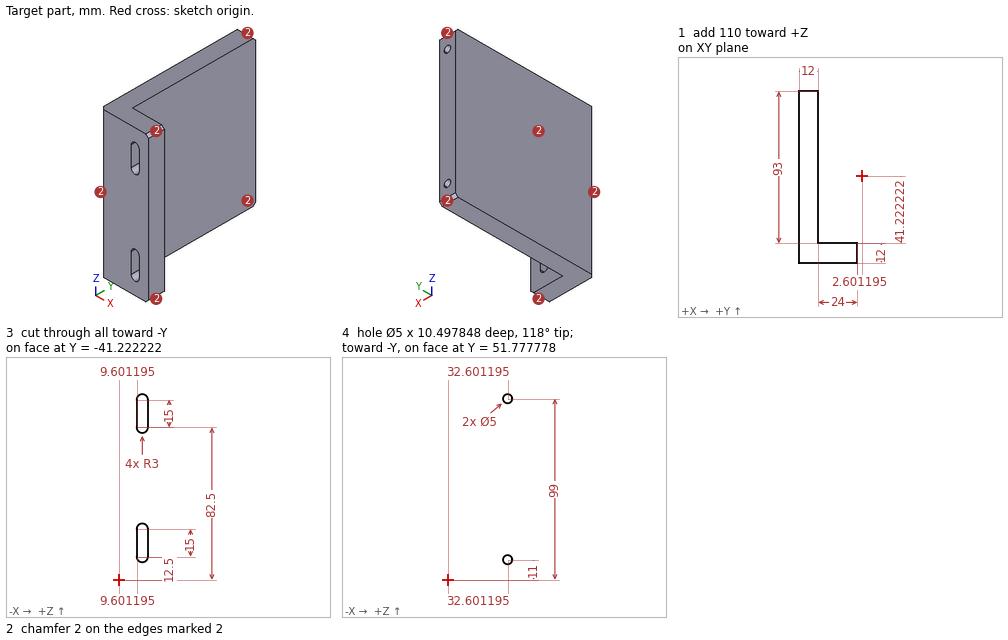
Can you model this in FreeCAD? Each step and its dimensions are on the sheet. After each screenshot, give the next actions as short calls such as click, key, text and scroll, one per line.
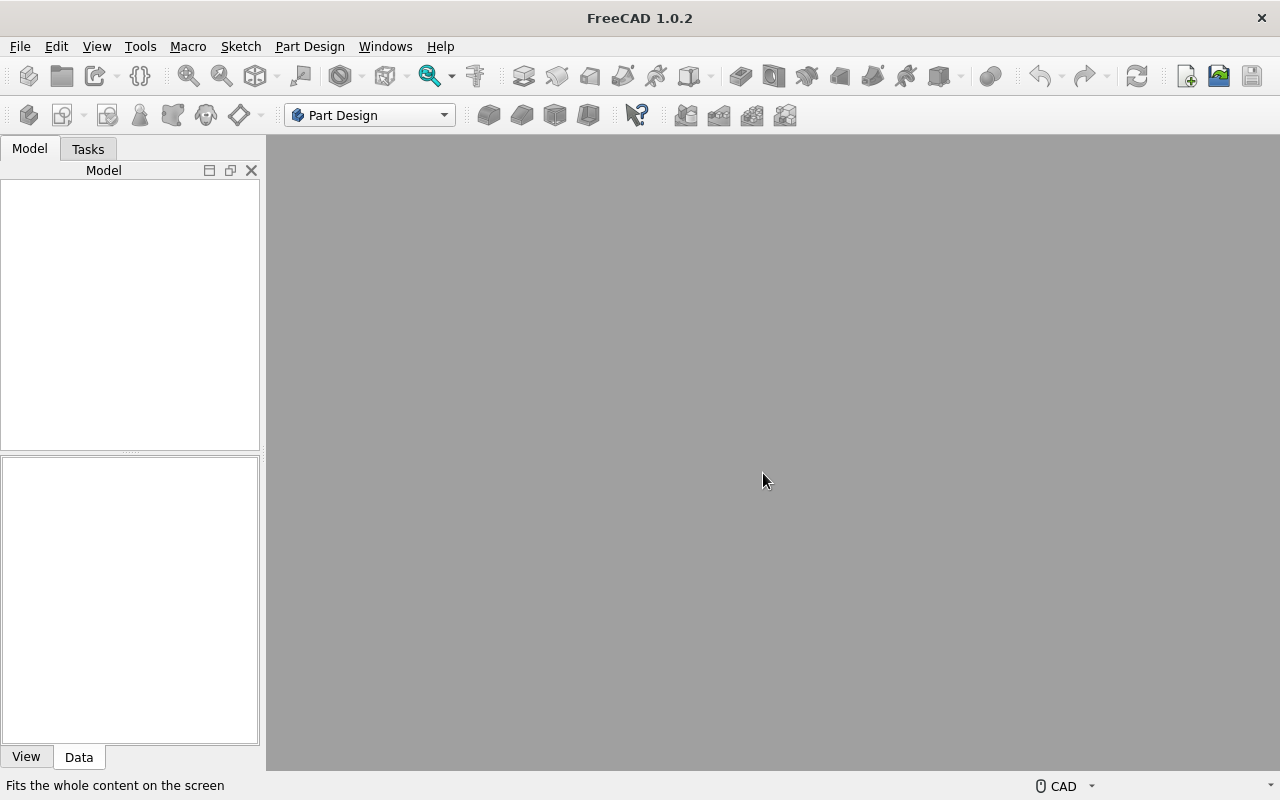
click(1186, 76)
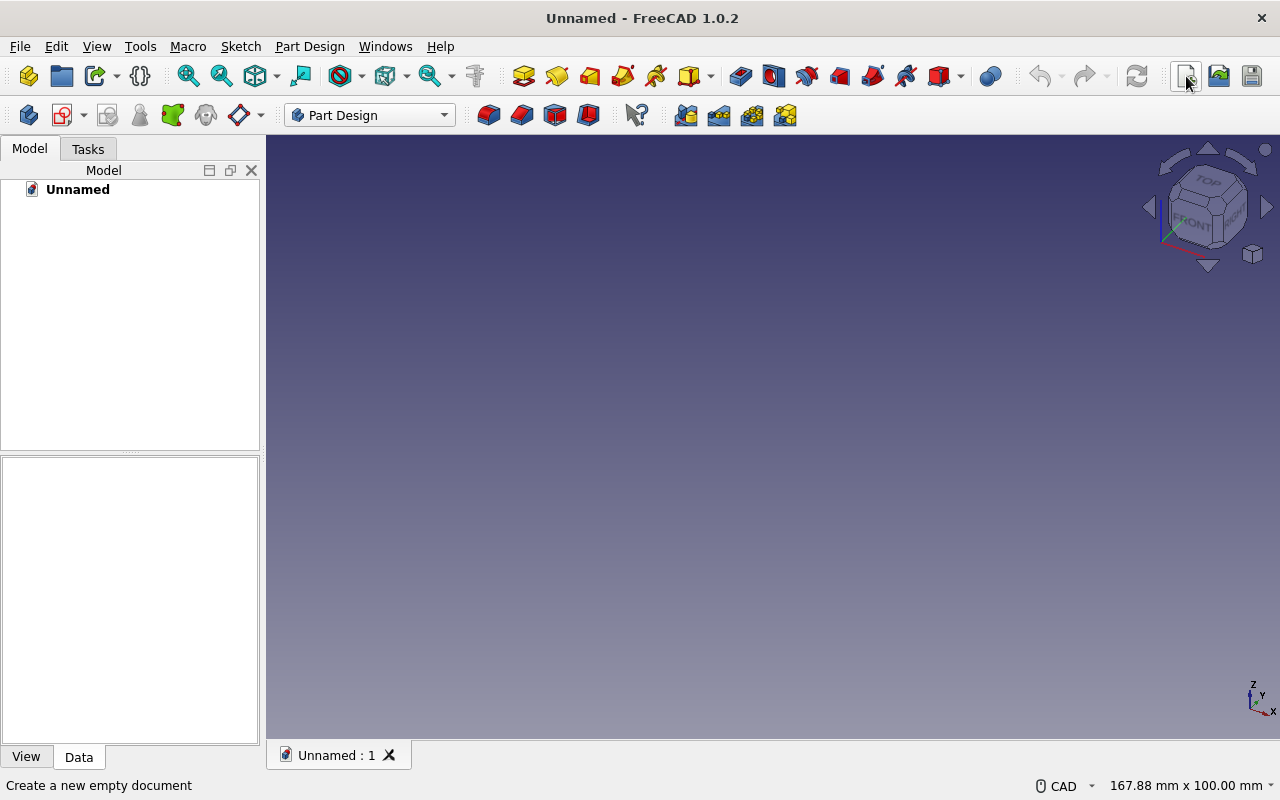
click(62, 116)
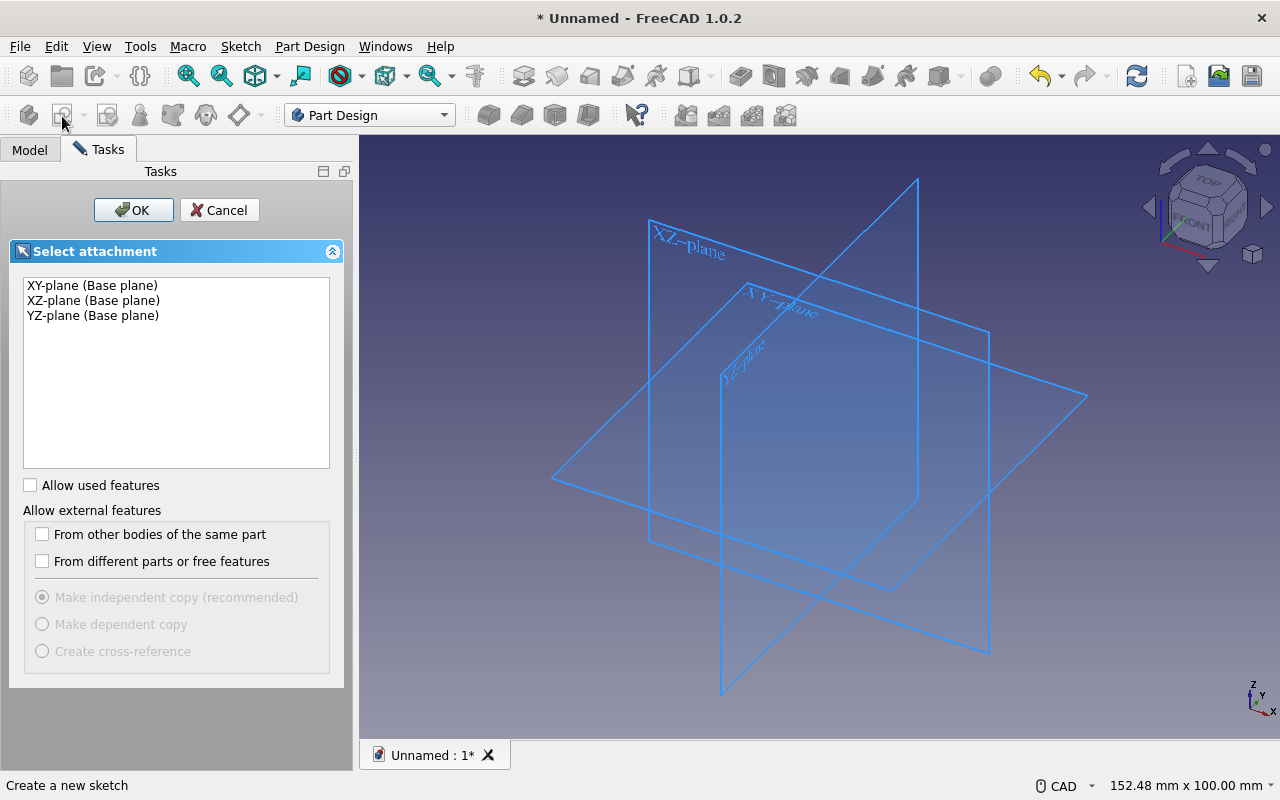
click(84, 286)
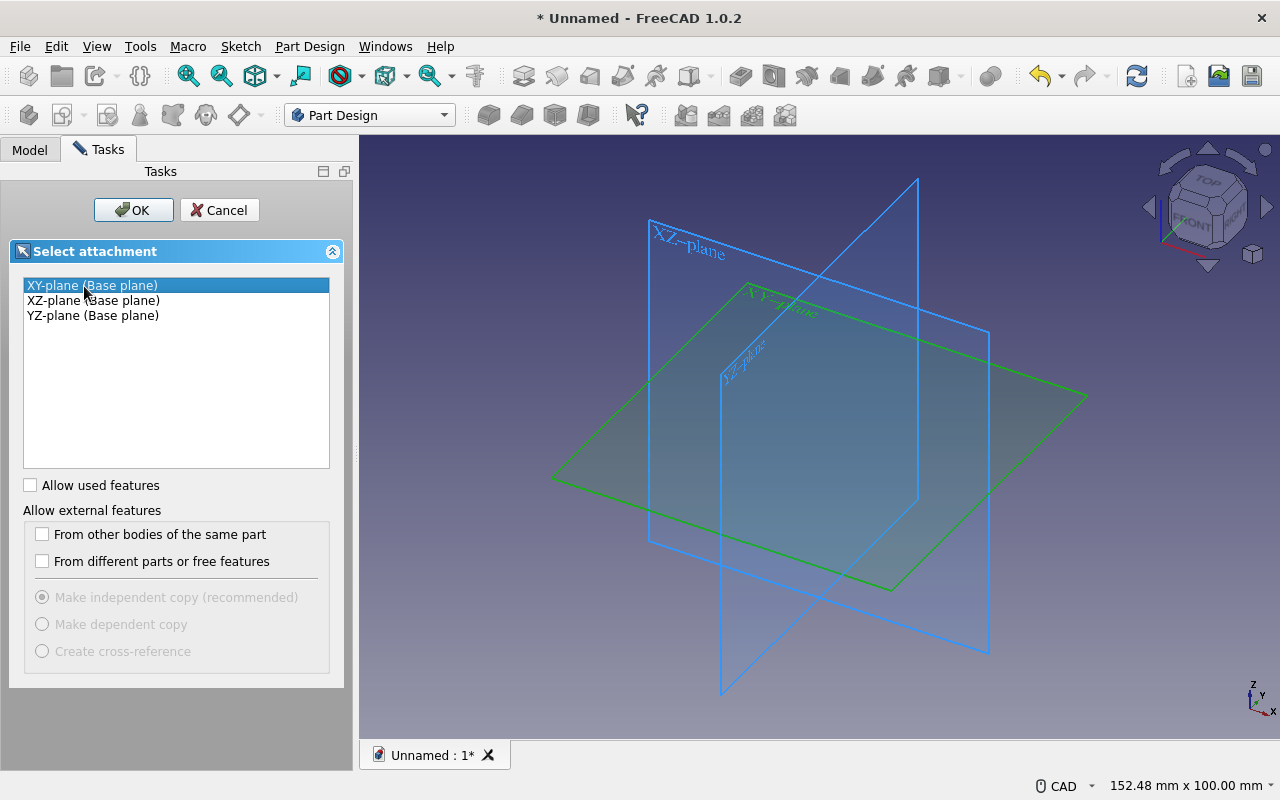
click(134, 210)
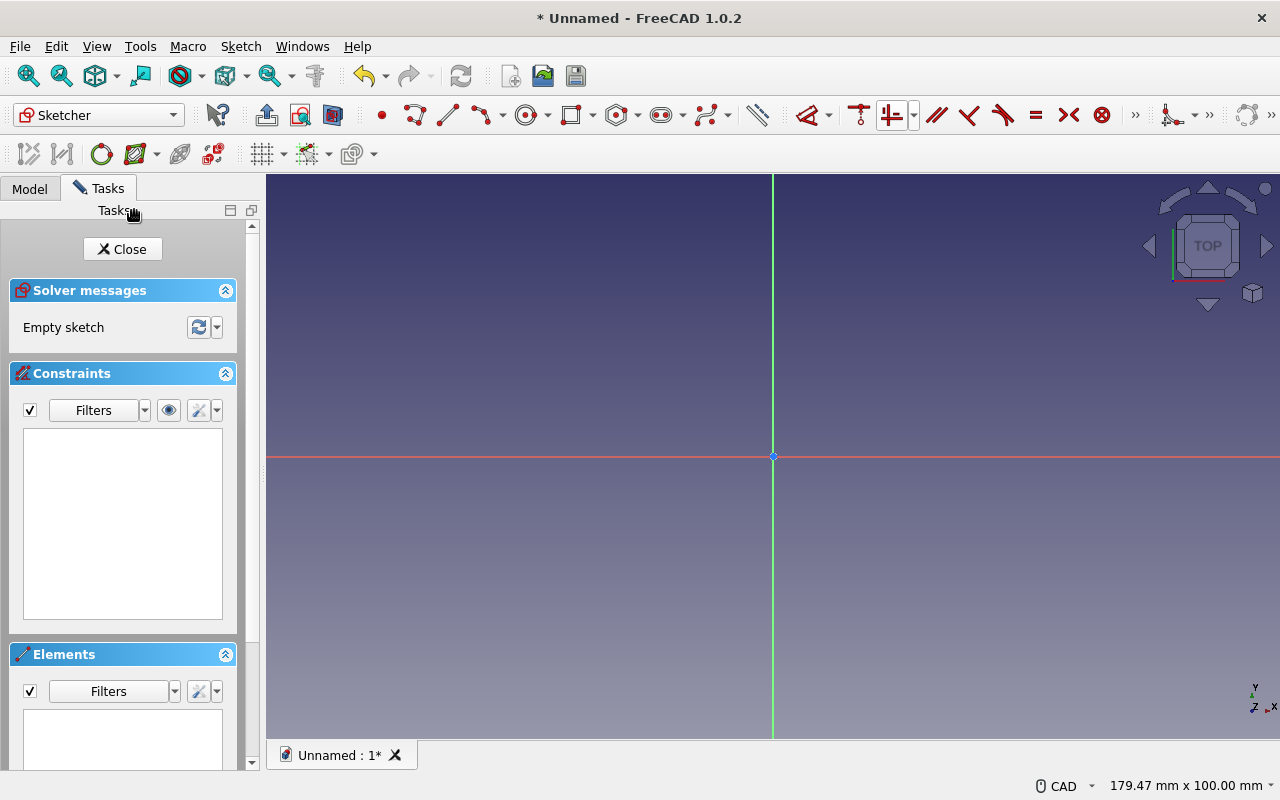
scroll(754, 452, down, 3)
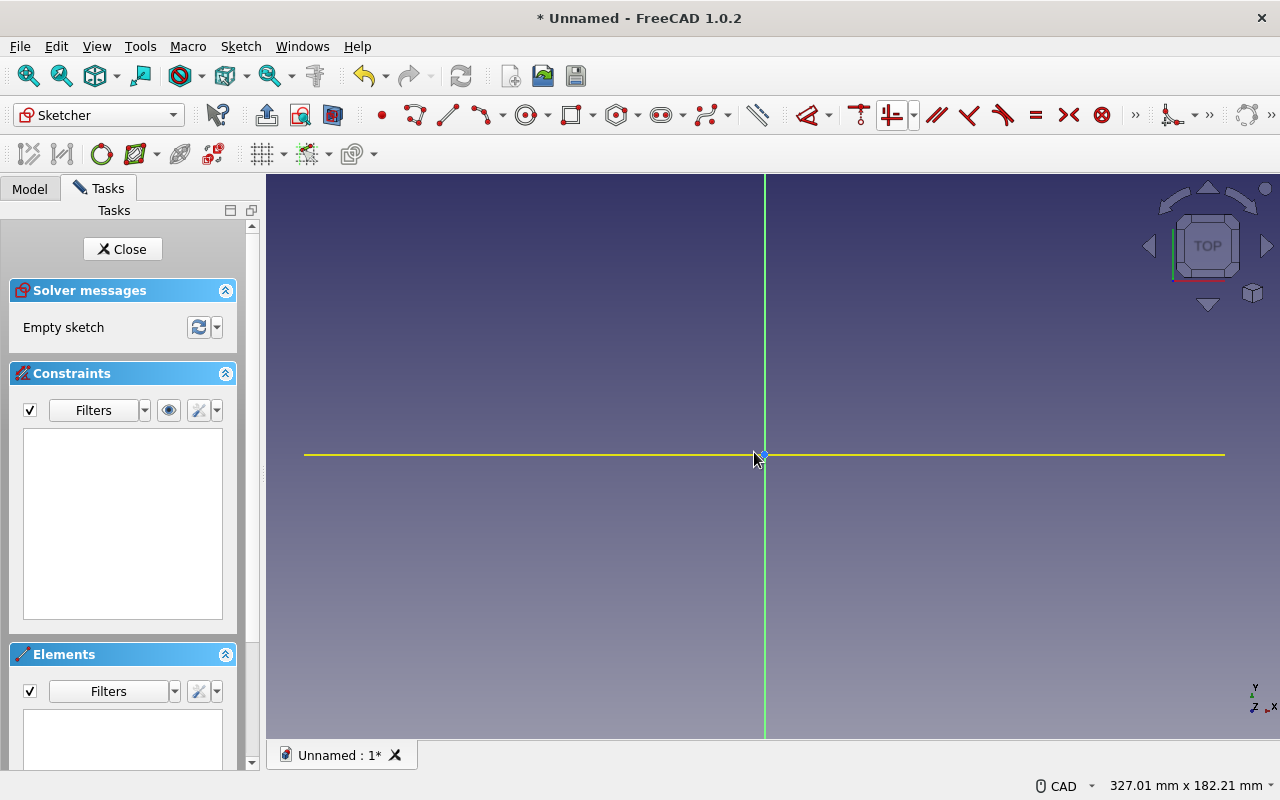
click(415, 116)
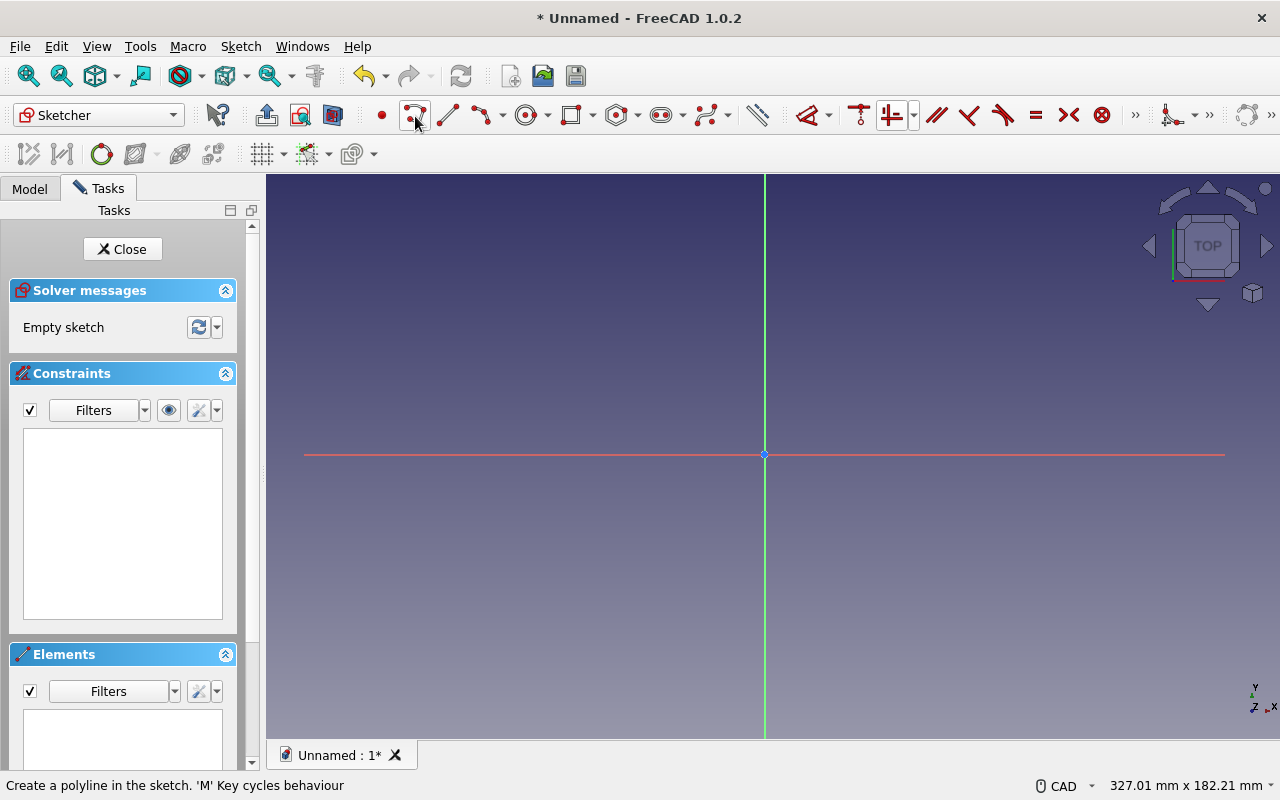
scroll(757, 583, up, 4)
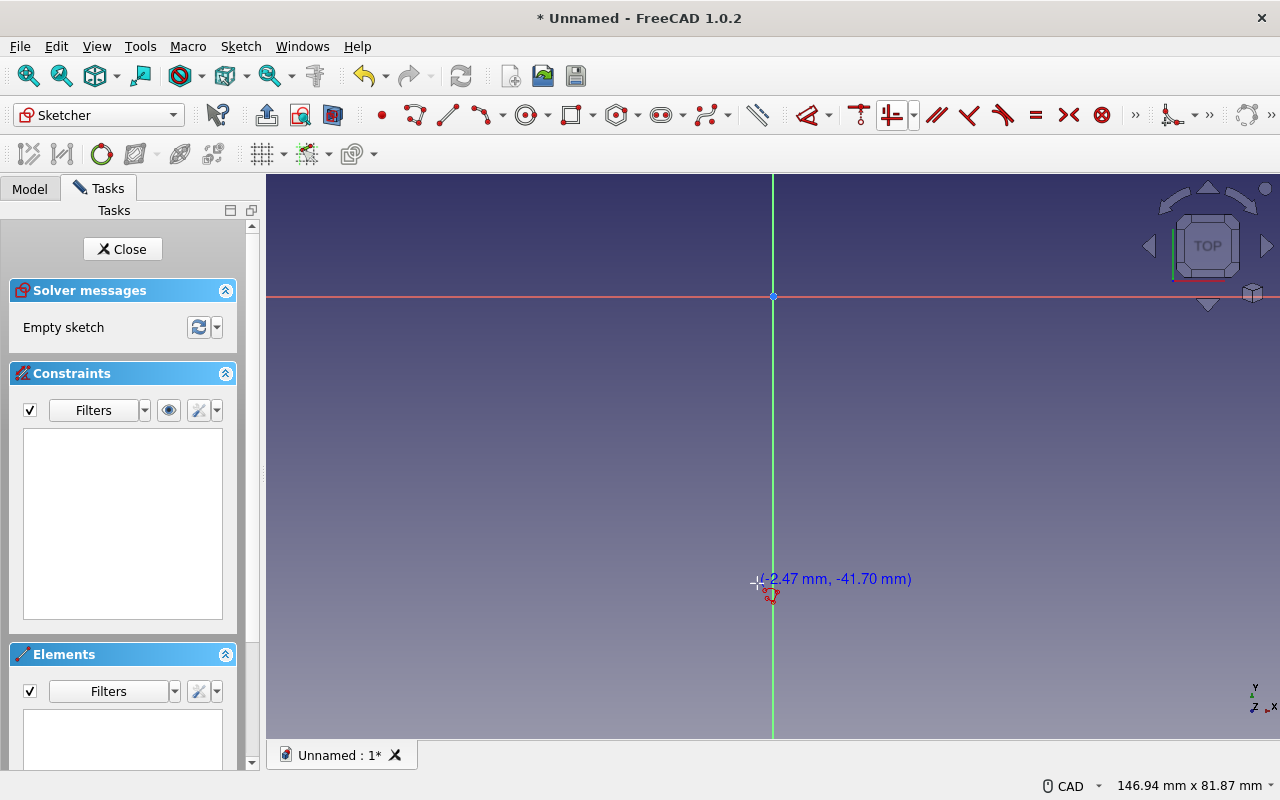
click(755, 581)
click(590, 581)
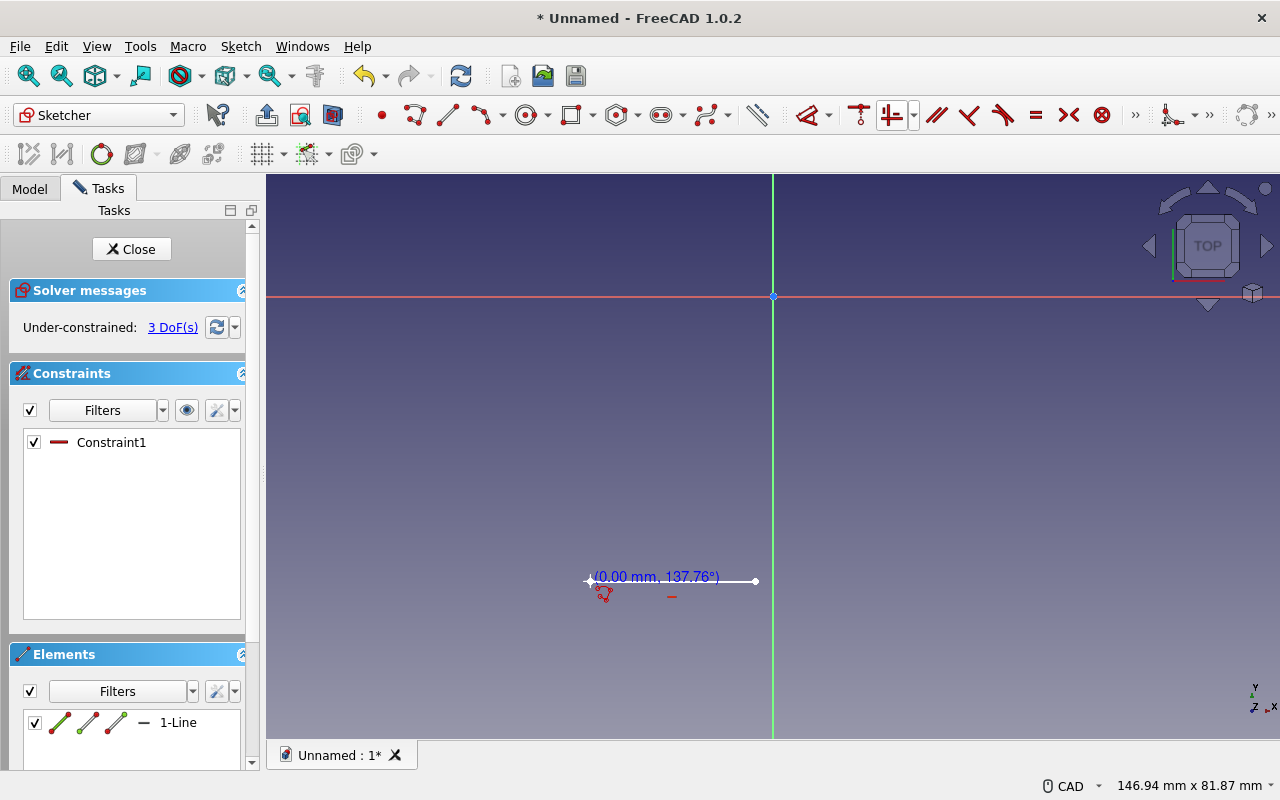
scroll(757, 583, down, 4)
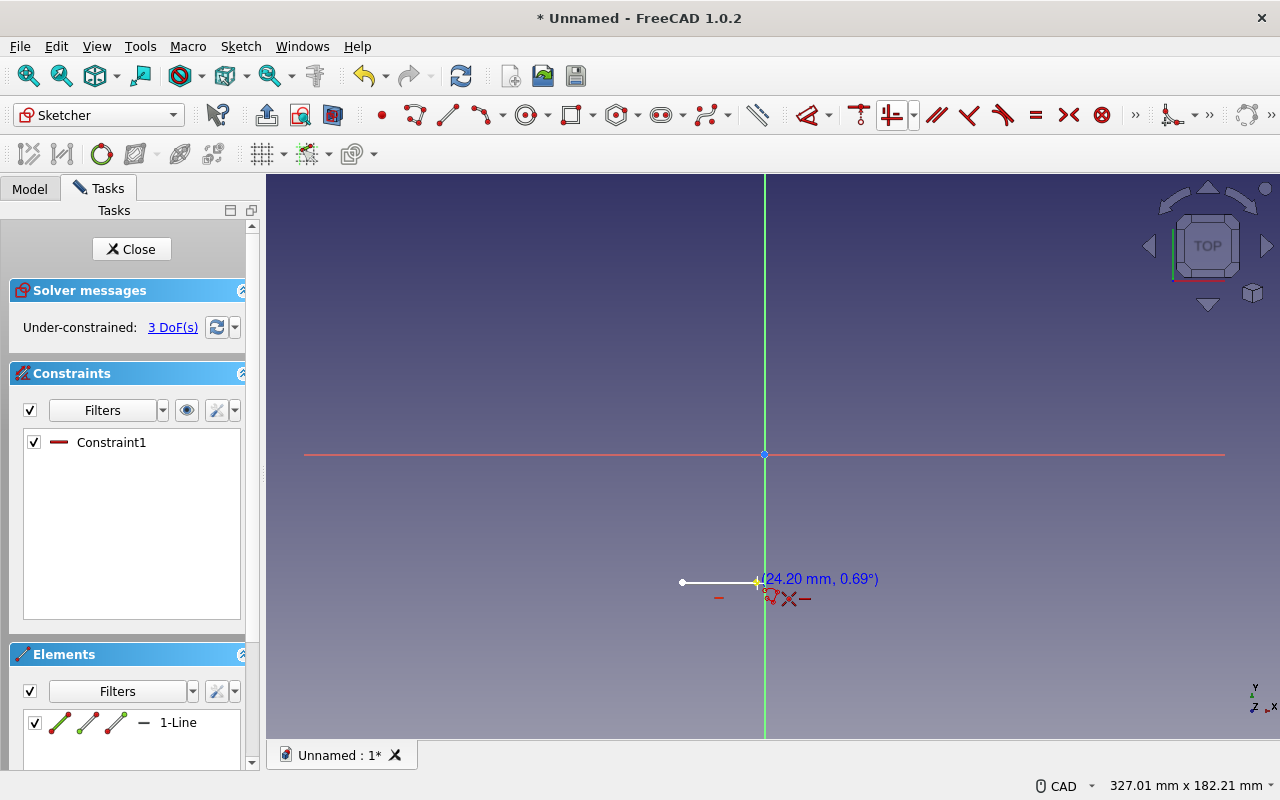
click(682, 294)
click(645, 294)
click(645, 620)